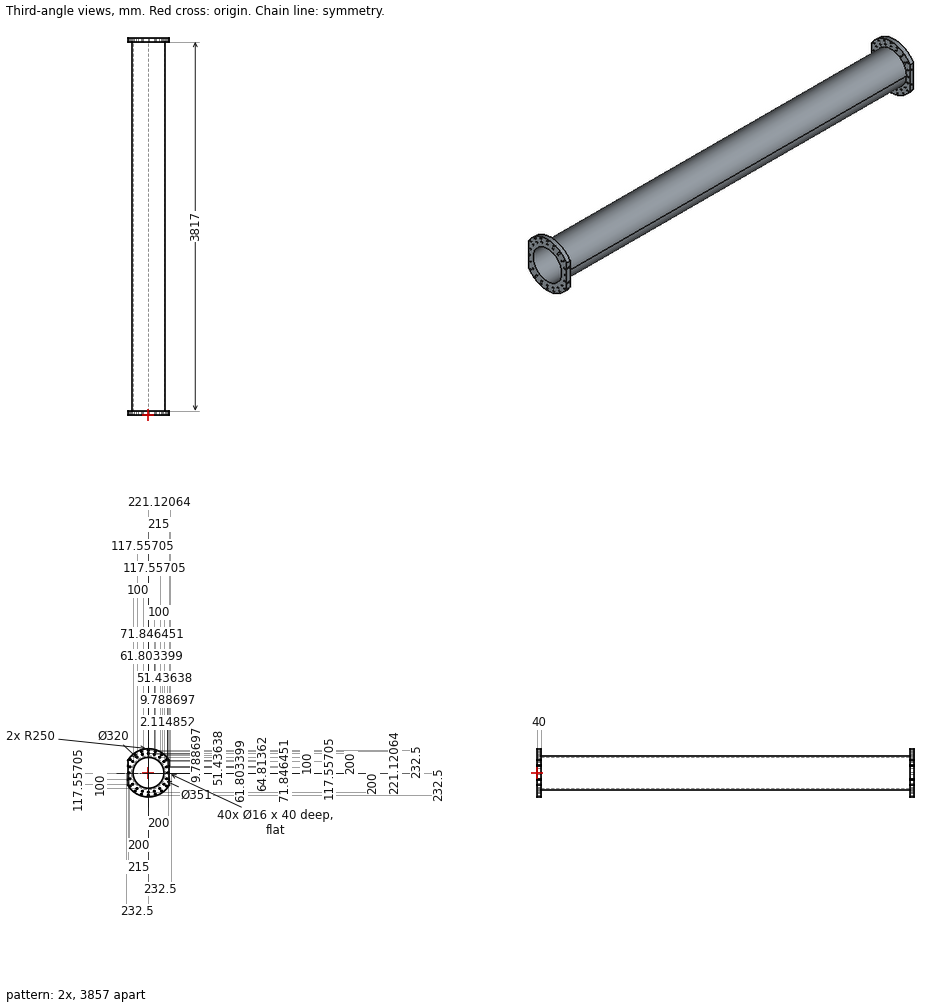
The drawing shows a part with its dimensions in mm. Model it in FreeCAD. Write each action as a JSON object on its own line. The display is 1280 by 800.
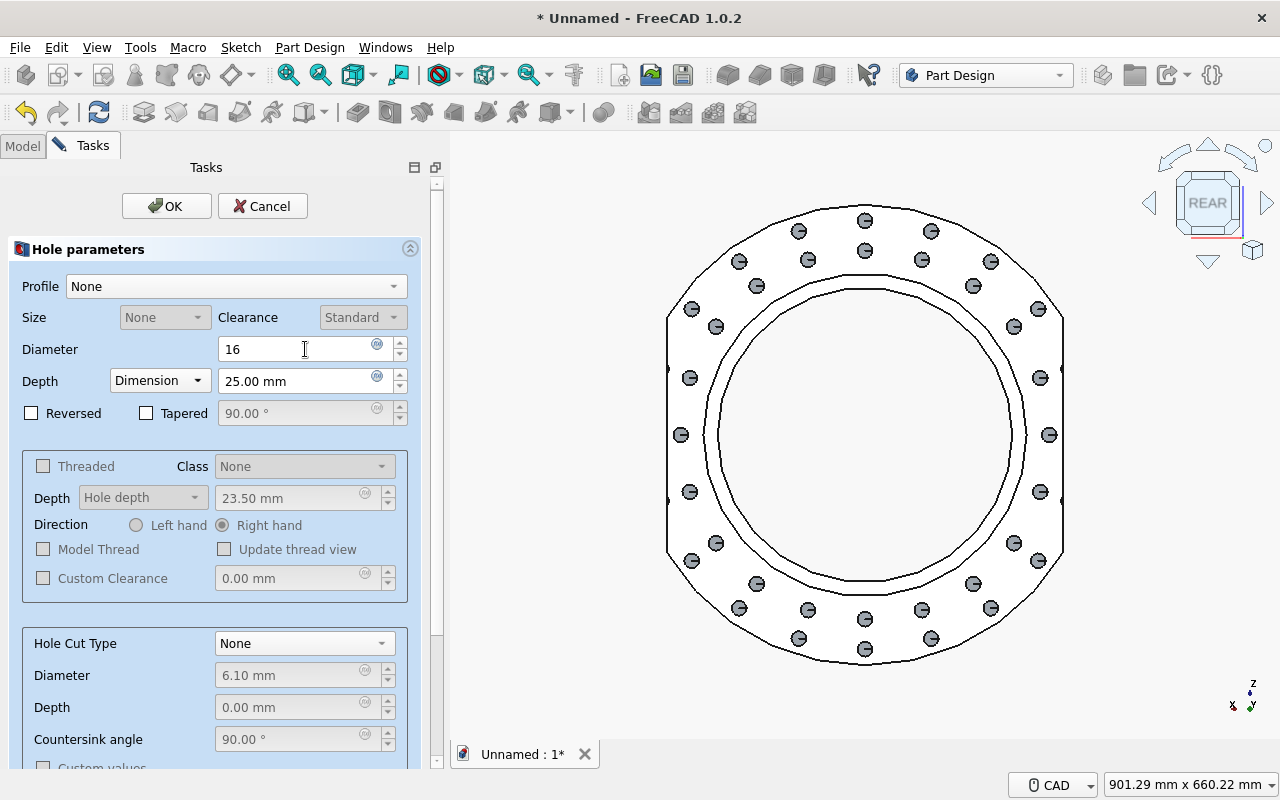
{"action": "triple_click", "coordinate": [305, 381]}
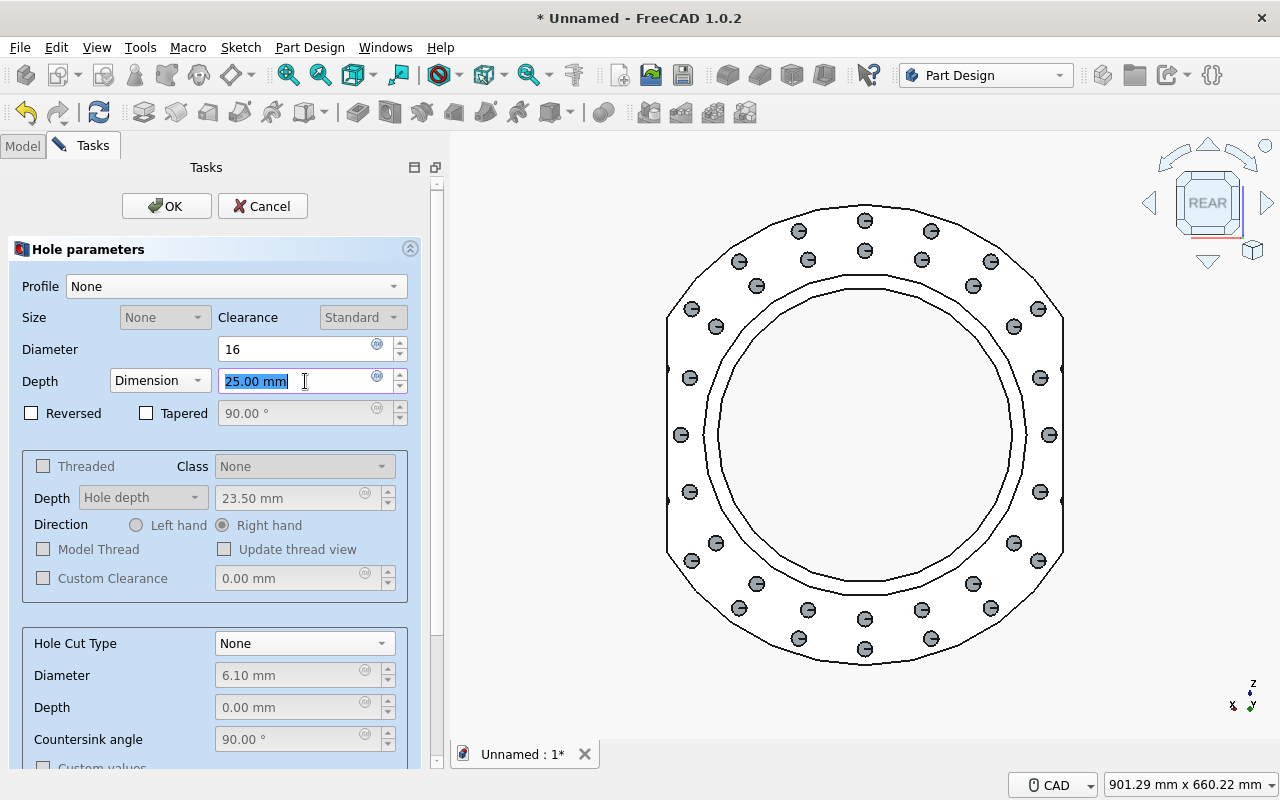
{"action": "type", "text": "40"}
{"action": "key", "text": "Tab"}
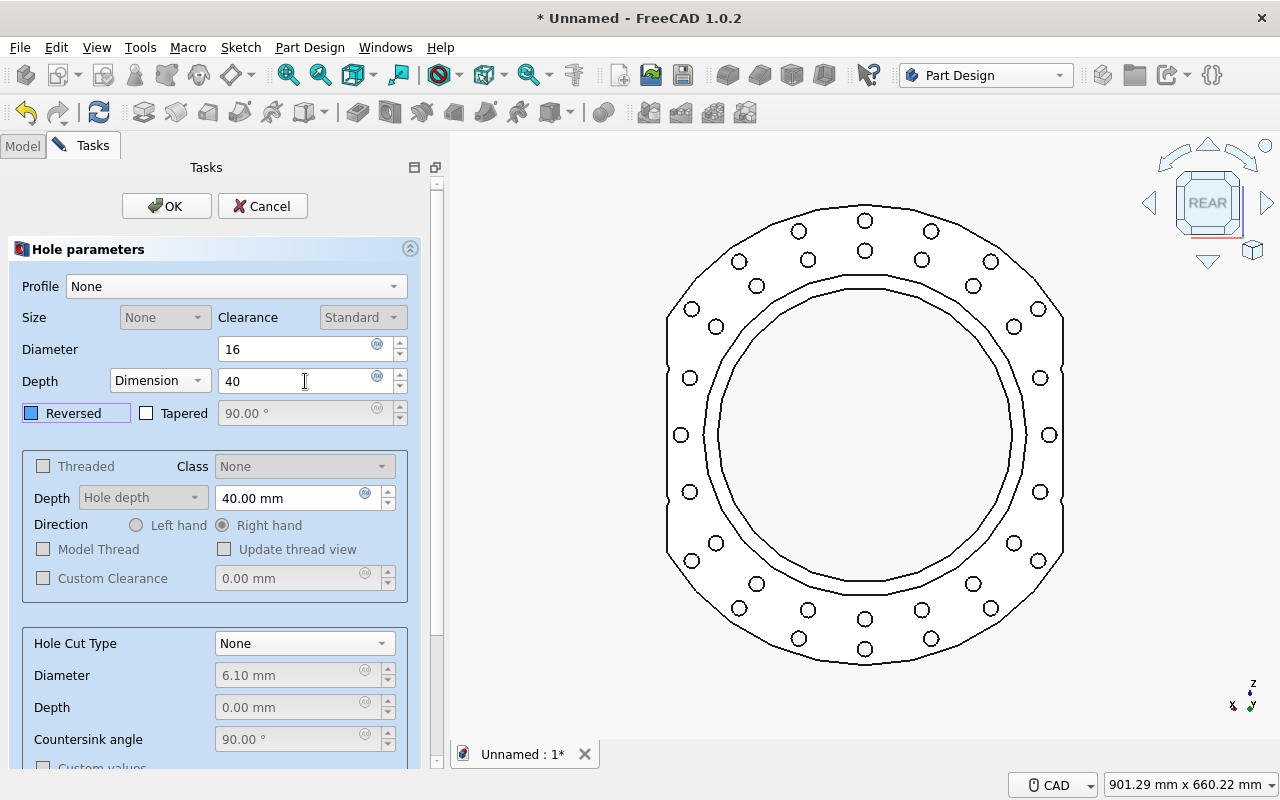
{"action": "scroll", "coordinate": [437, 472], "scroll_direction": "down", "scroll_amount": 3}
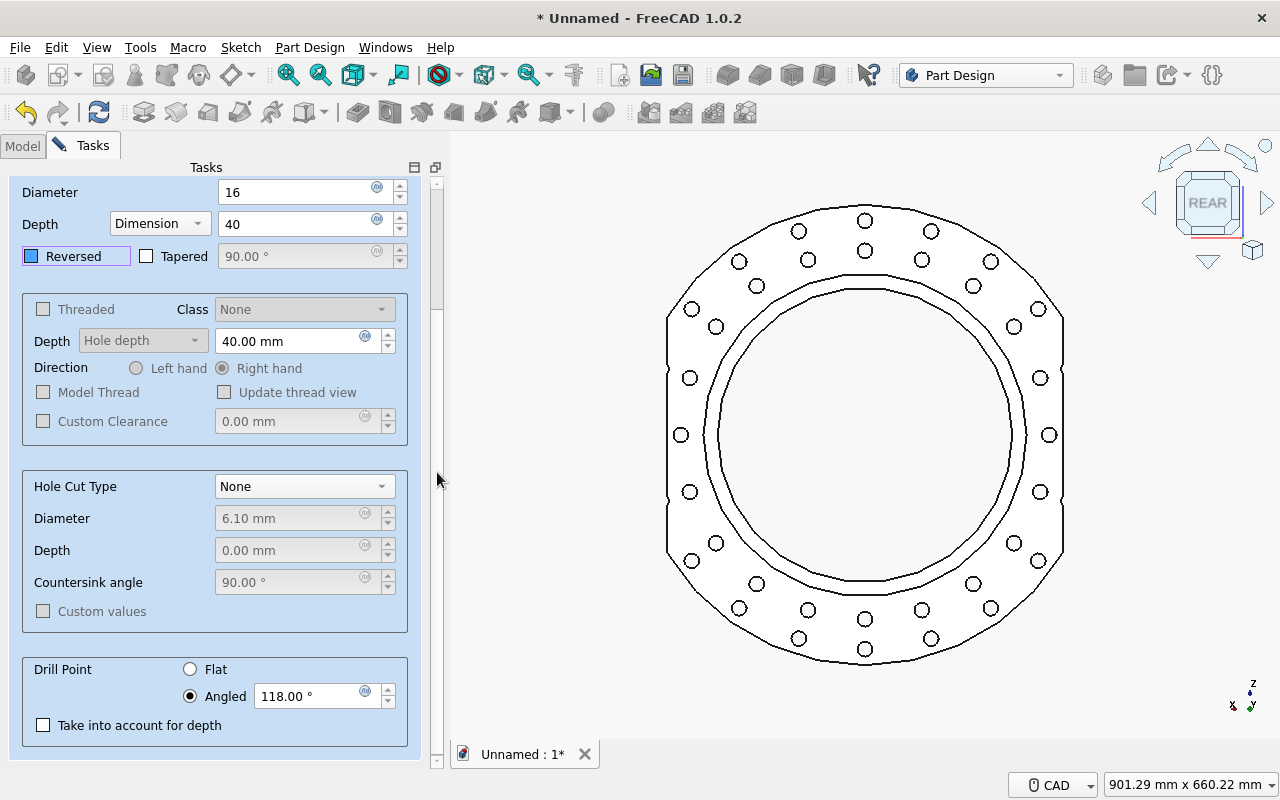
{"action": "left_click", "coordinate": [191, 669]}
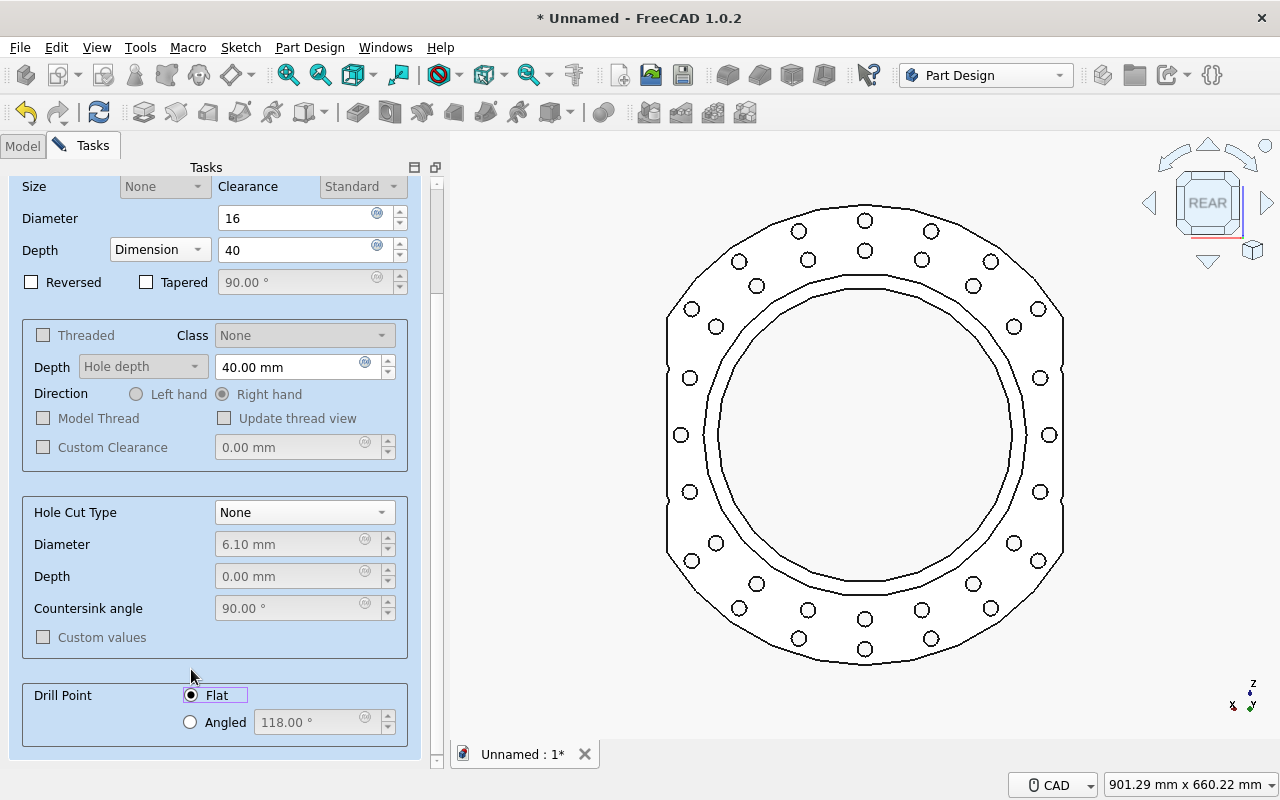
{"action": "scroll", "coordinate": [437, 472], "scroll_direction": "up", "scroll_amount": 3}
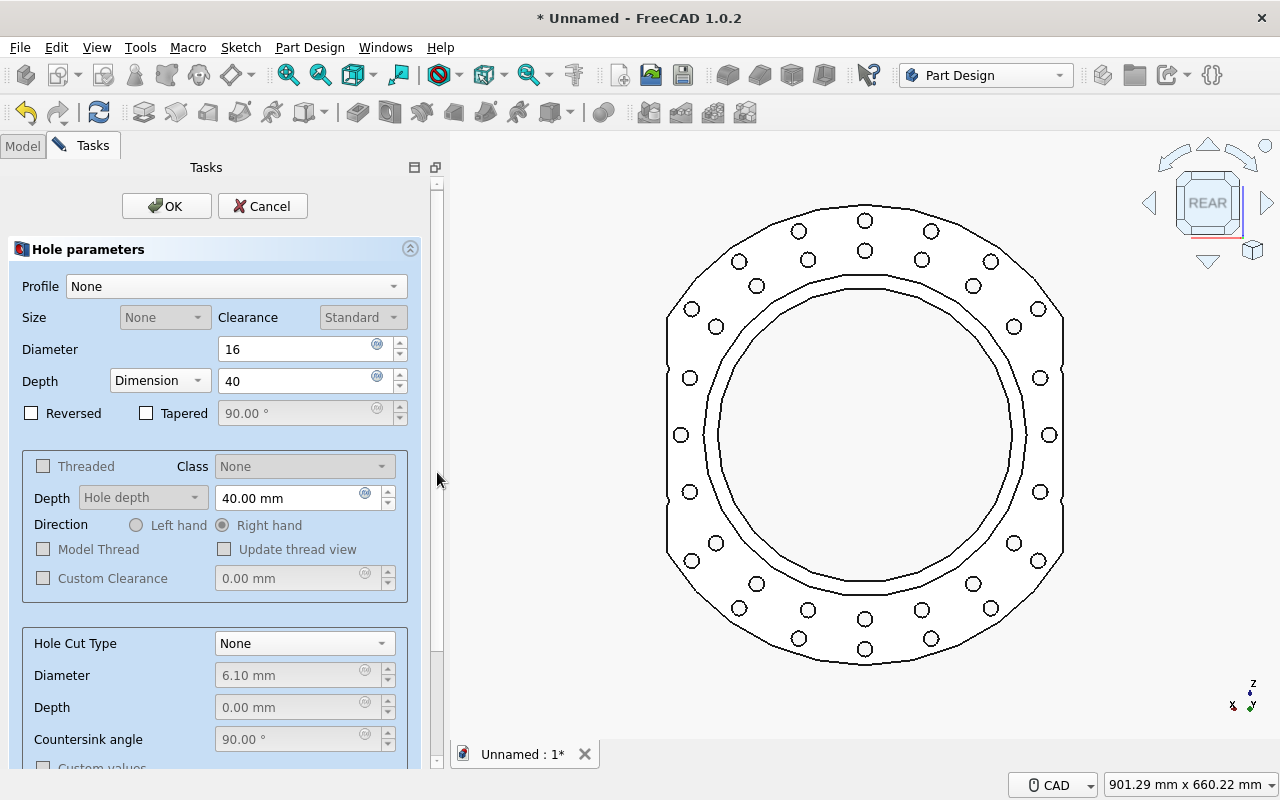
{"action": "left_click", "coordinate": [167, 206]}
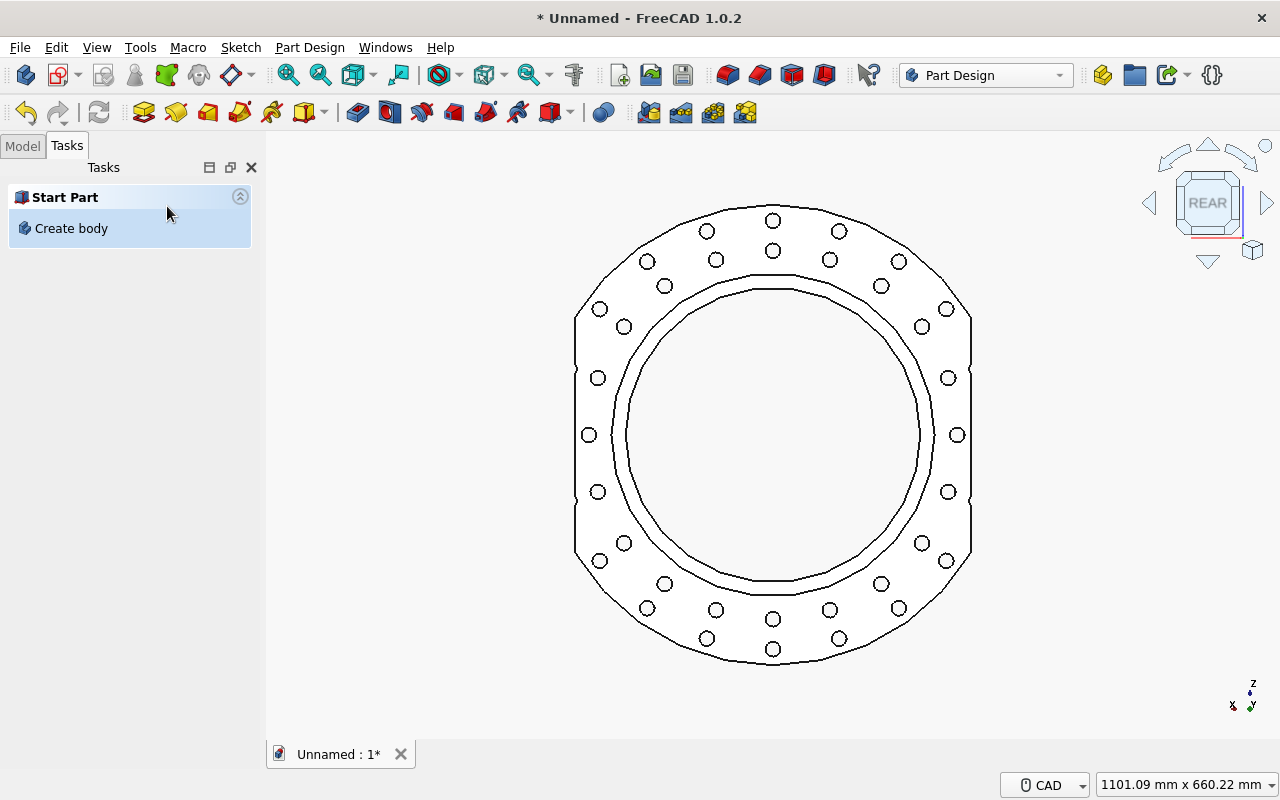
{"action": "left_click", "coordinate": [23, 145]}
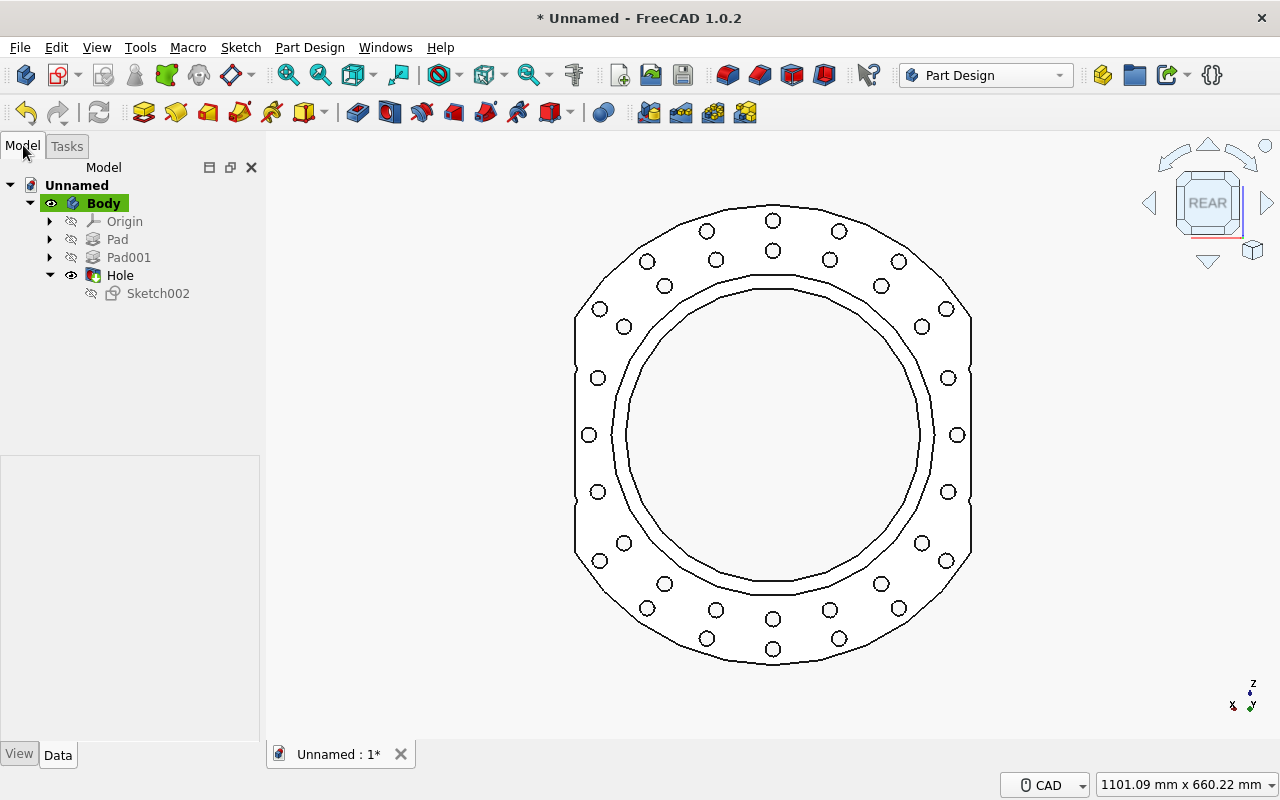
{"action": "left_click", "coordinate": [116, 239]}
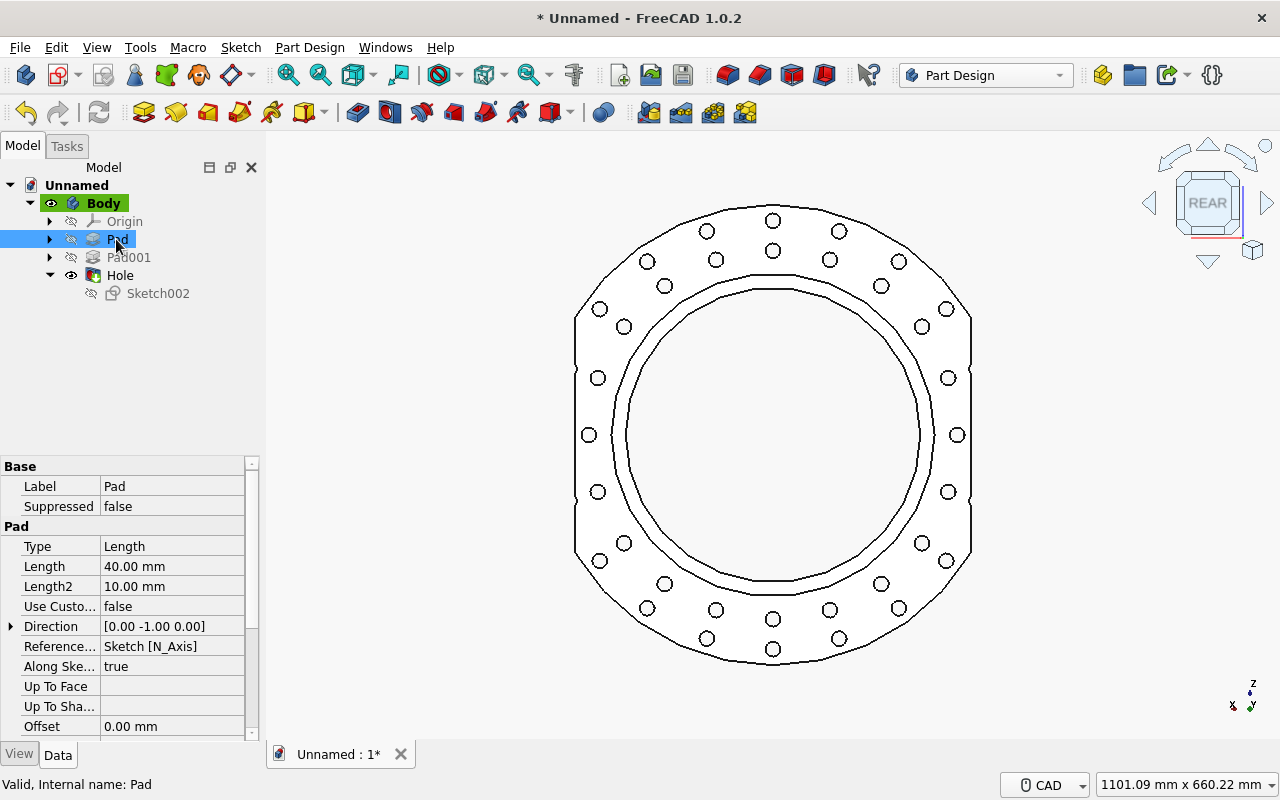
{"action": "left_click", "coordinate": [116, 275], "text": "ctrl"}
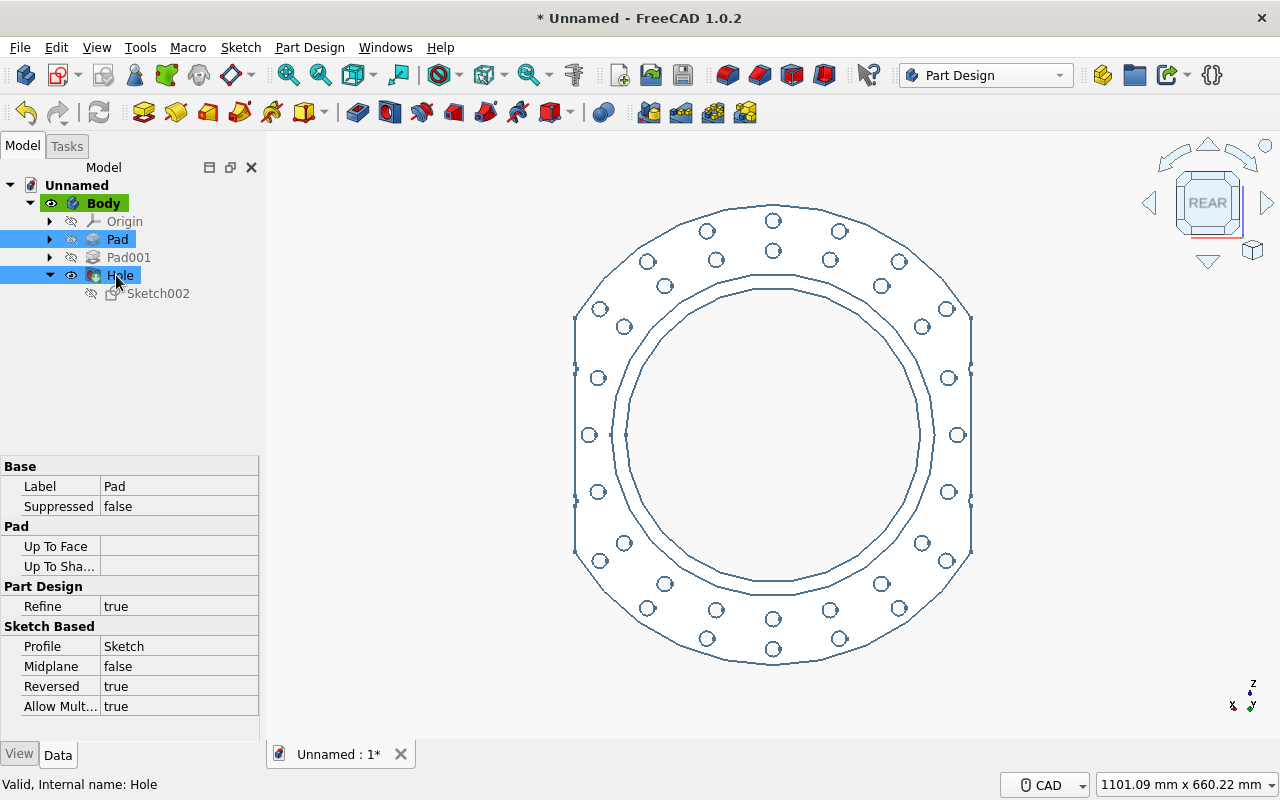
{"action": "left_click", "coordinate": [682, 112]}